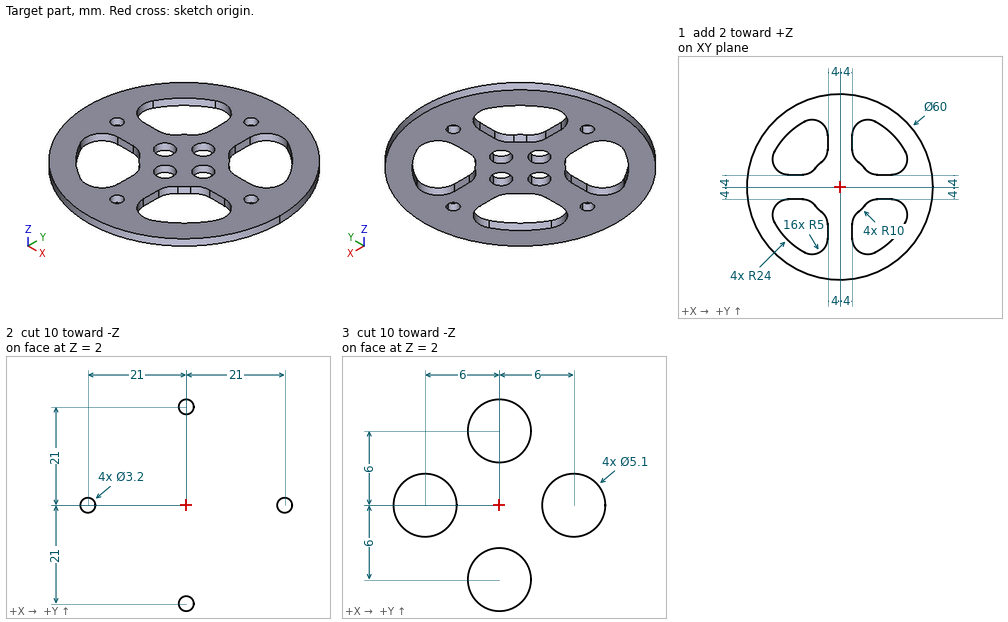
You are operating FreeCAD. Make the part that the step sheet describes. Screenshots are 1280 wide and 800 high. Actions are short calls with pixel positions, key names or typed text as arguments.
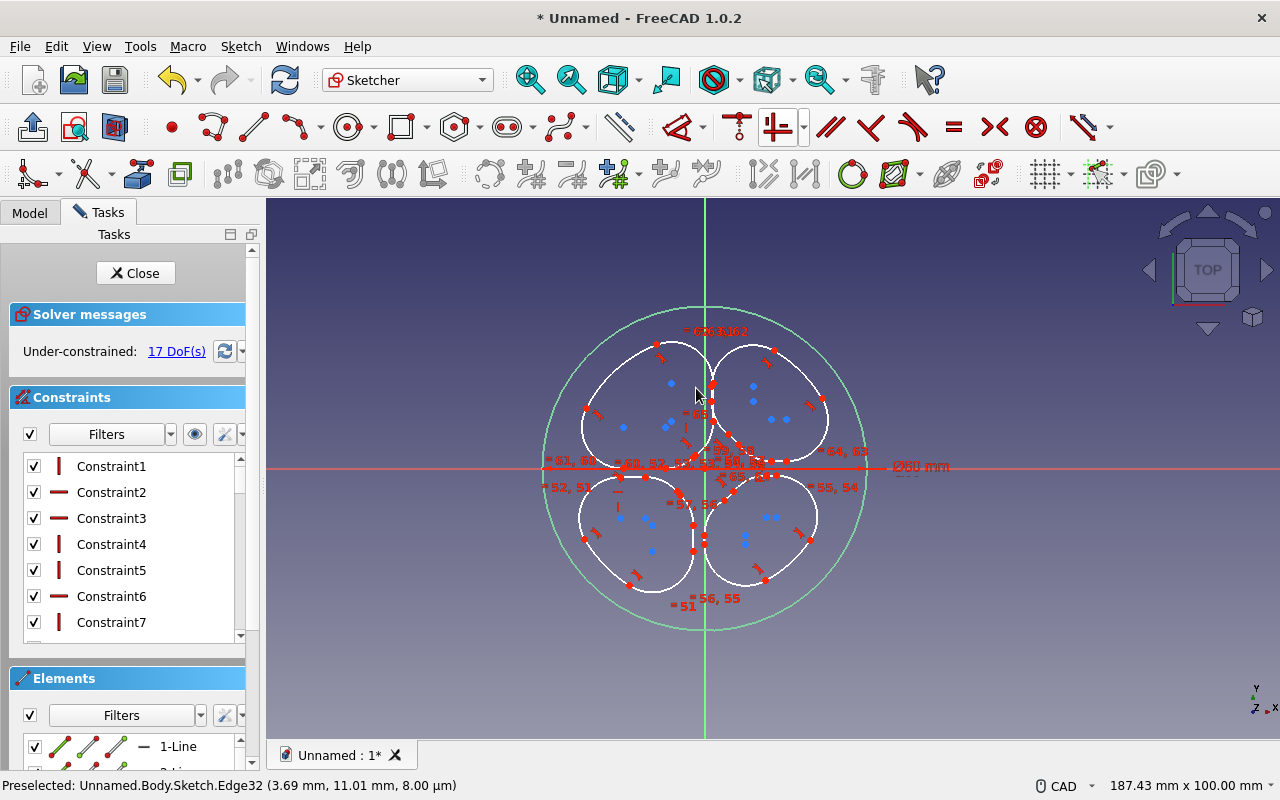
click(596, 556)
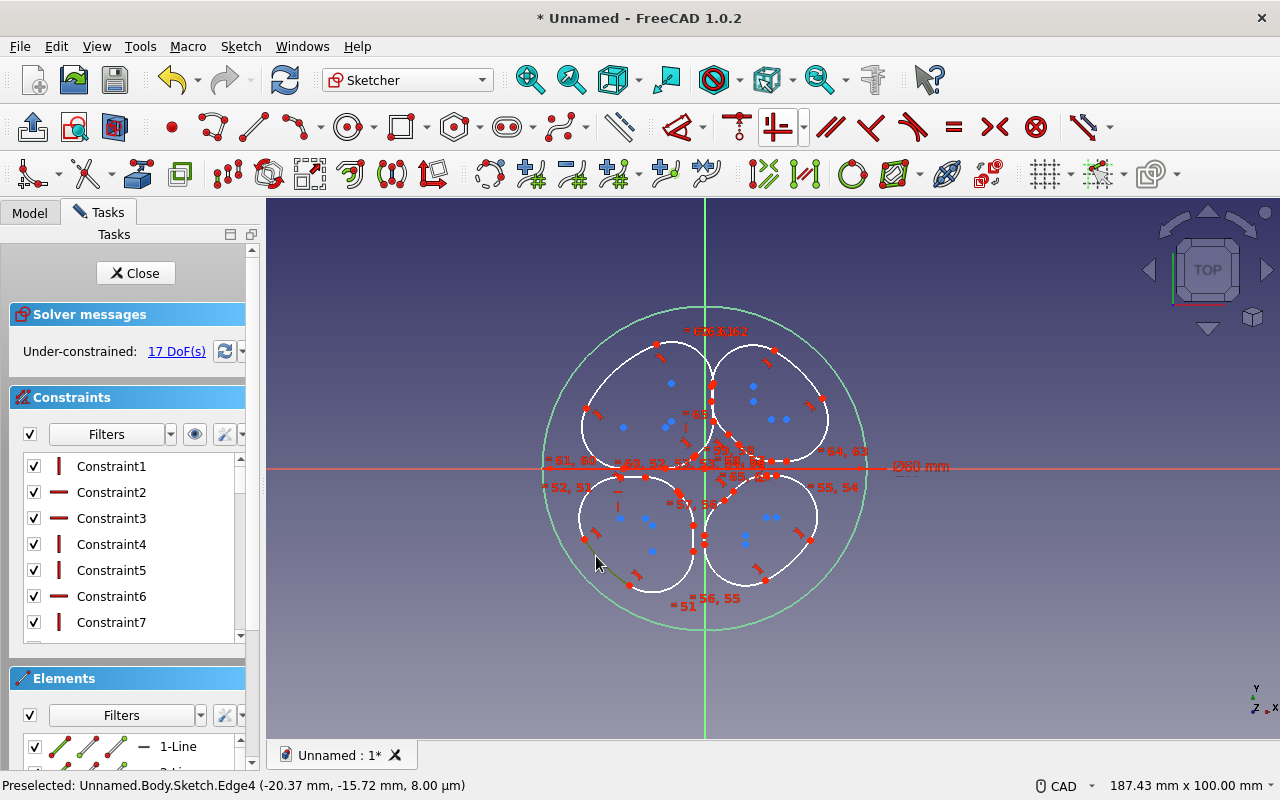
click(781, 571)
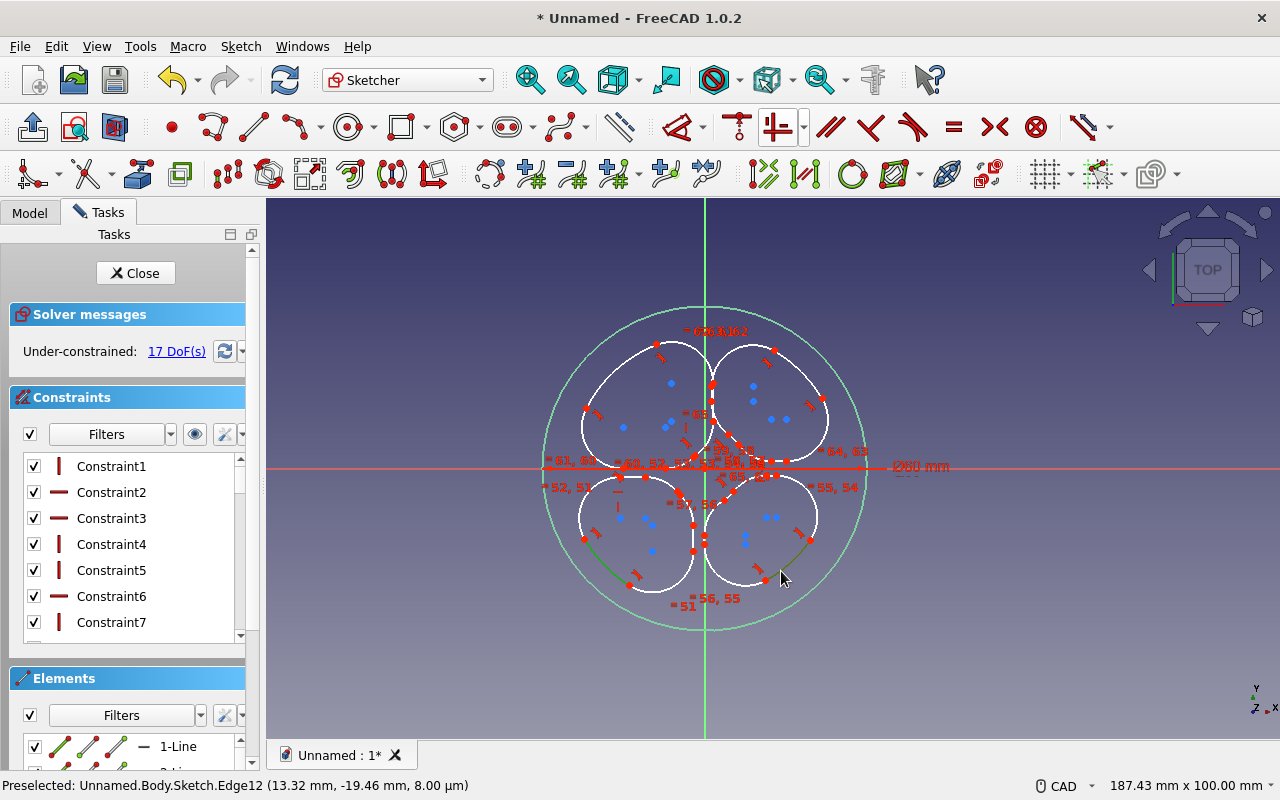
click(631, 358)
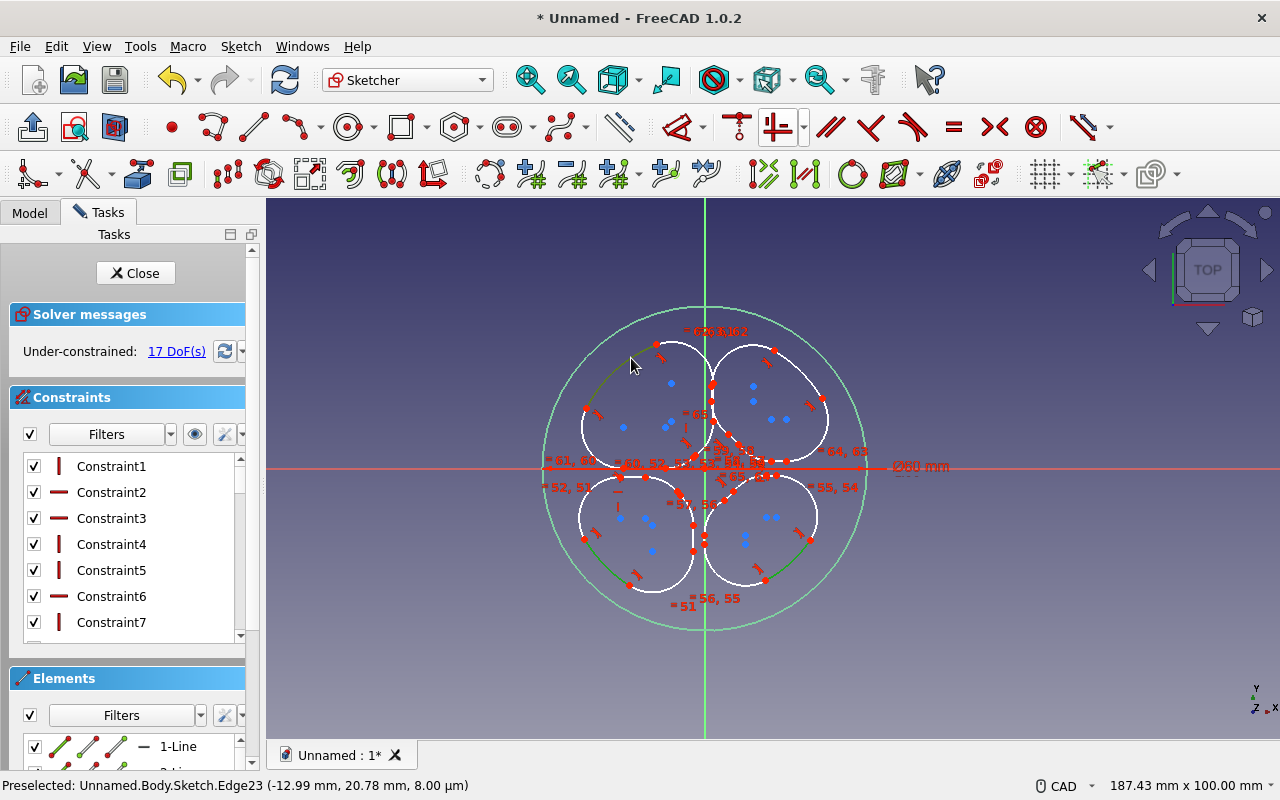
click(810, 382)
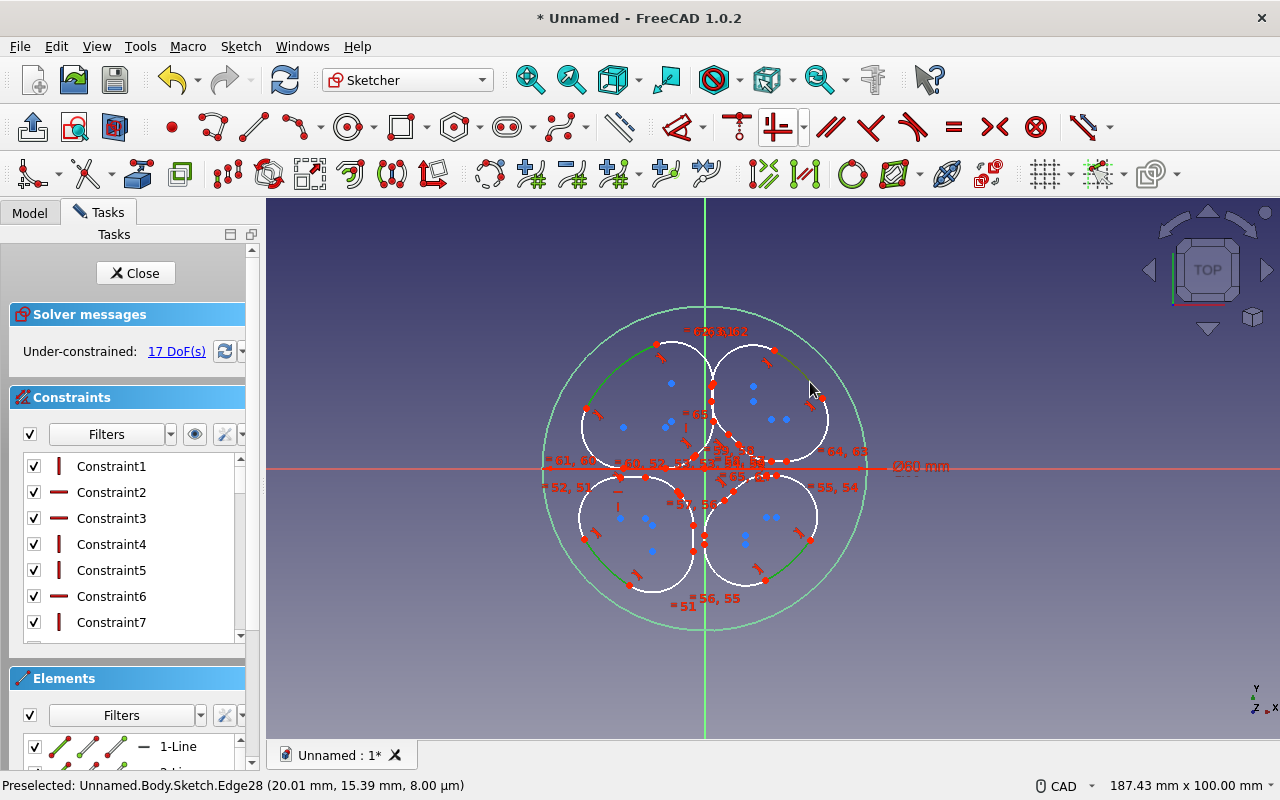
key(e)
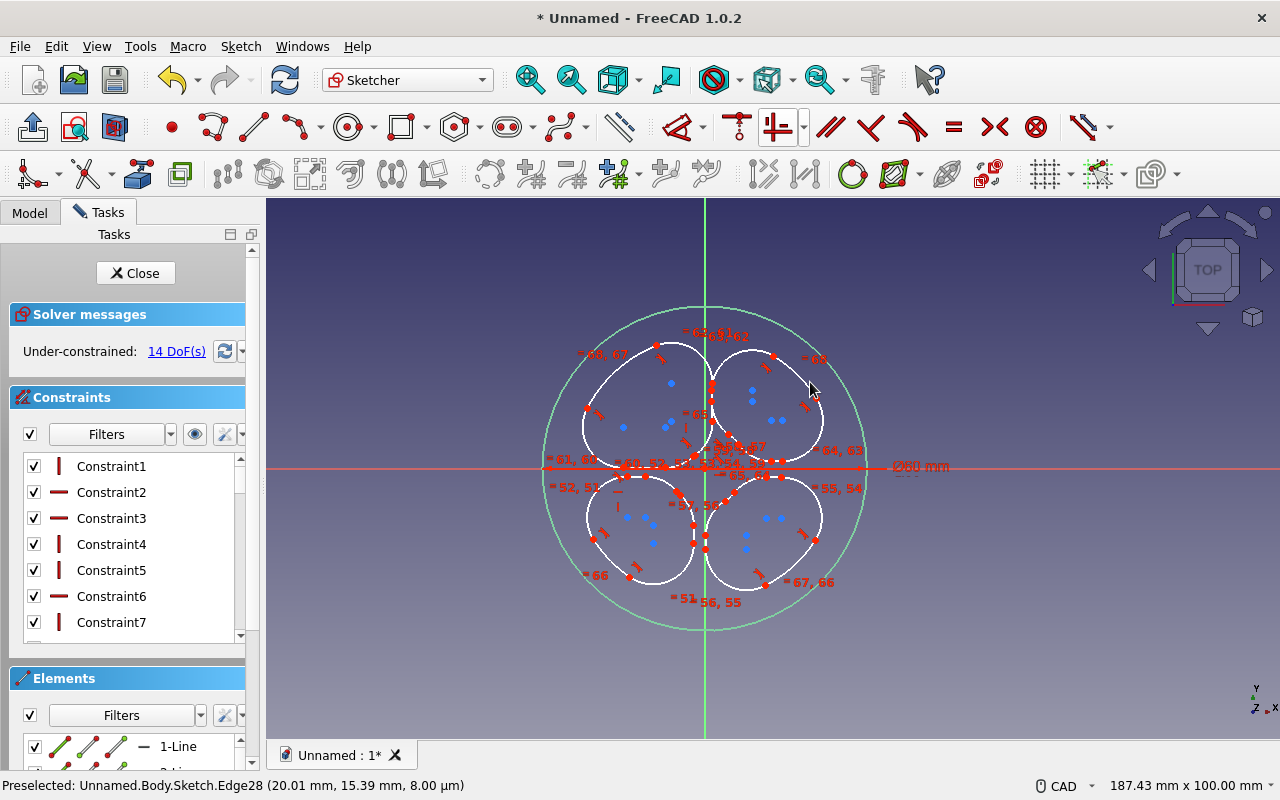
scroll(679, 493, up, 9)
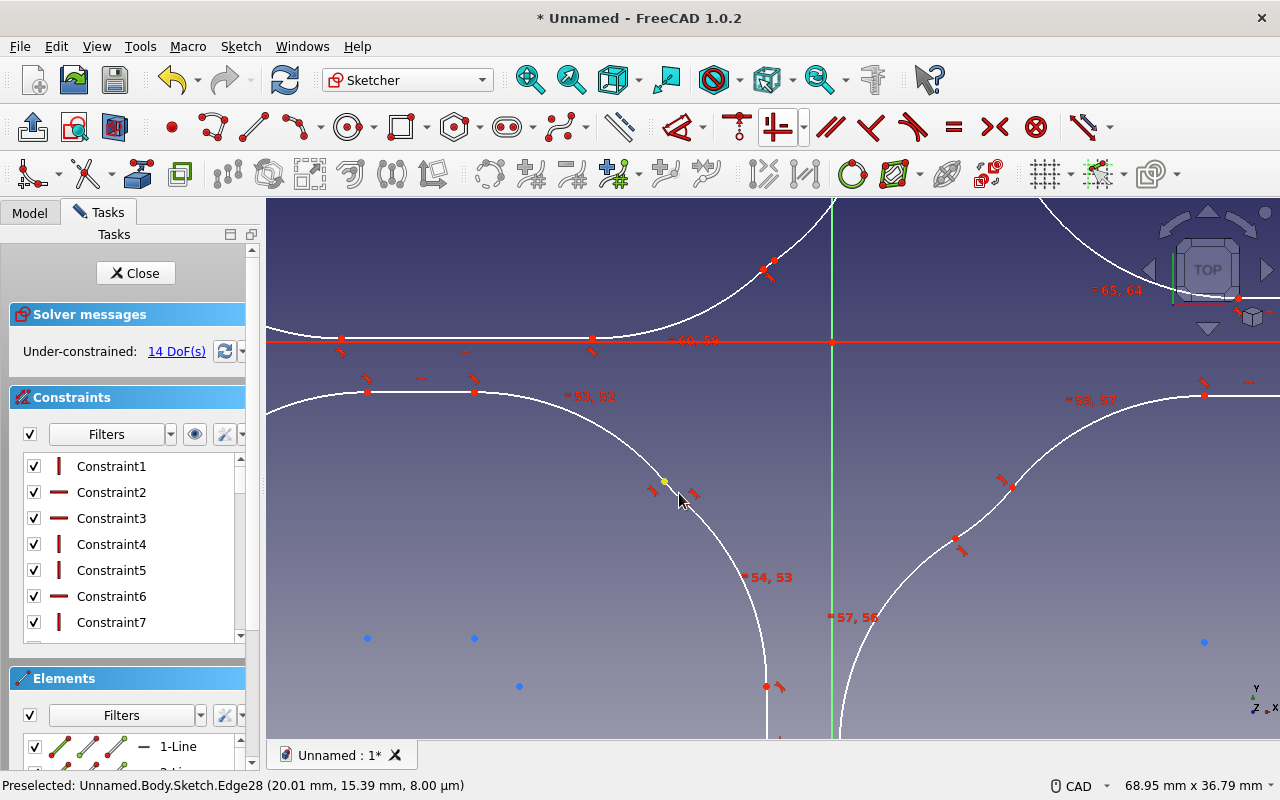
click(675, 493)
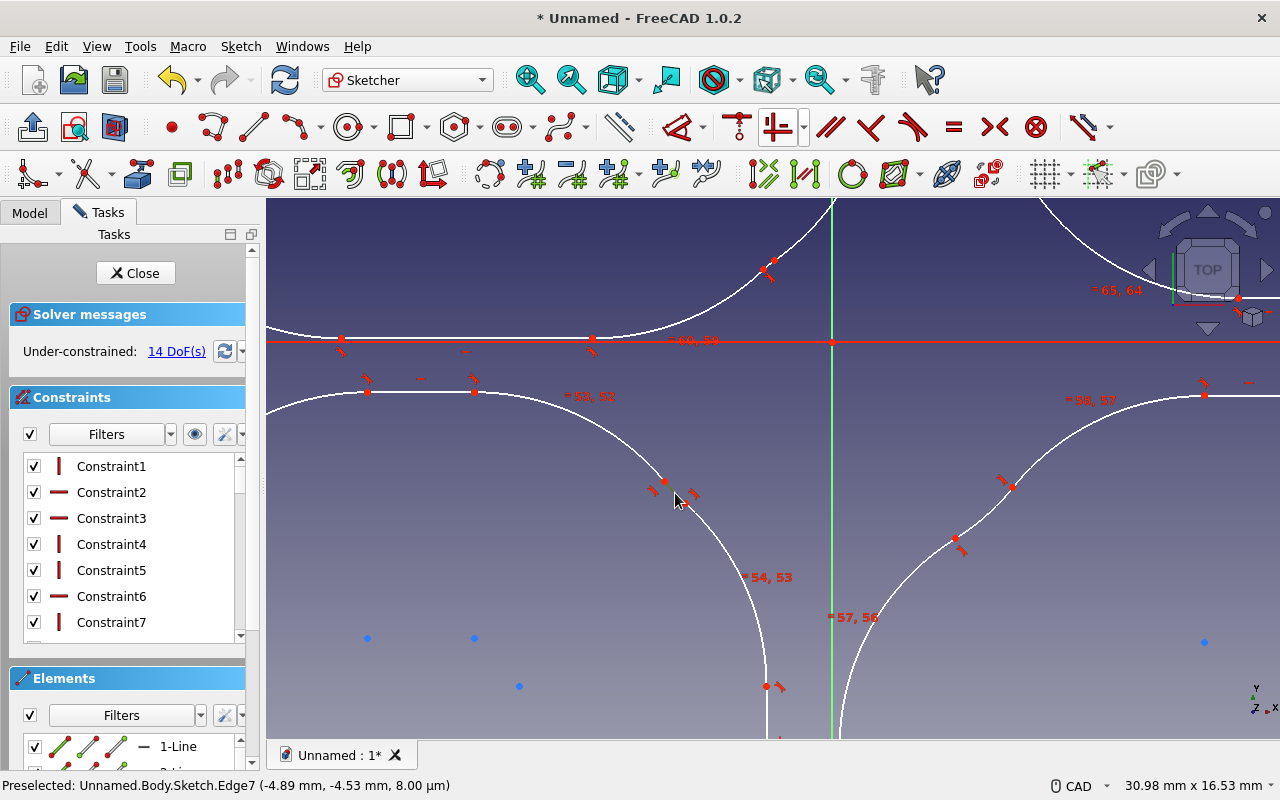
click(974, 525)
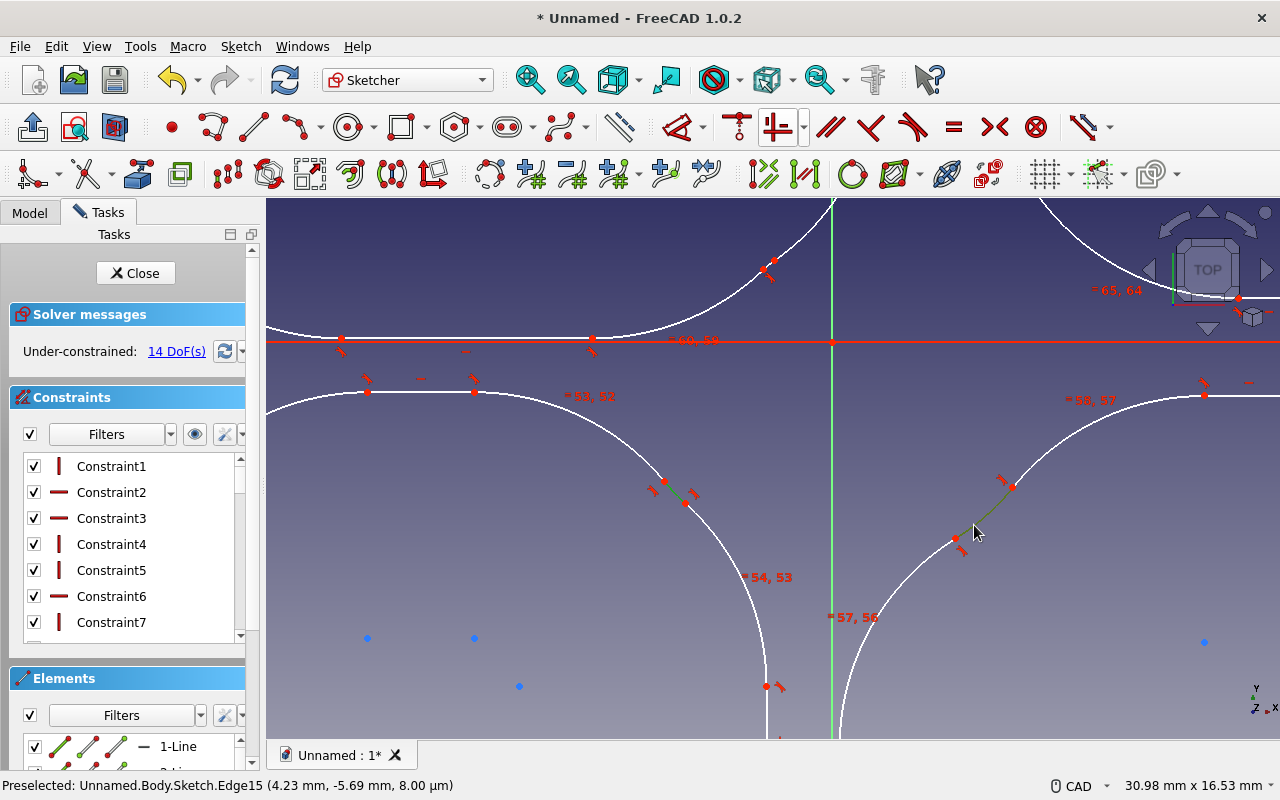
scroll(769, 265, up, 4)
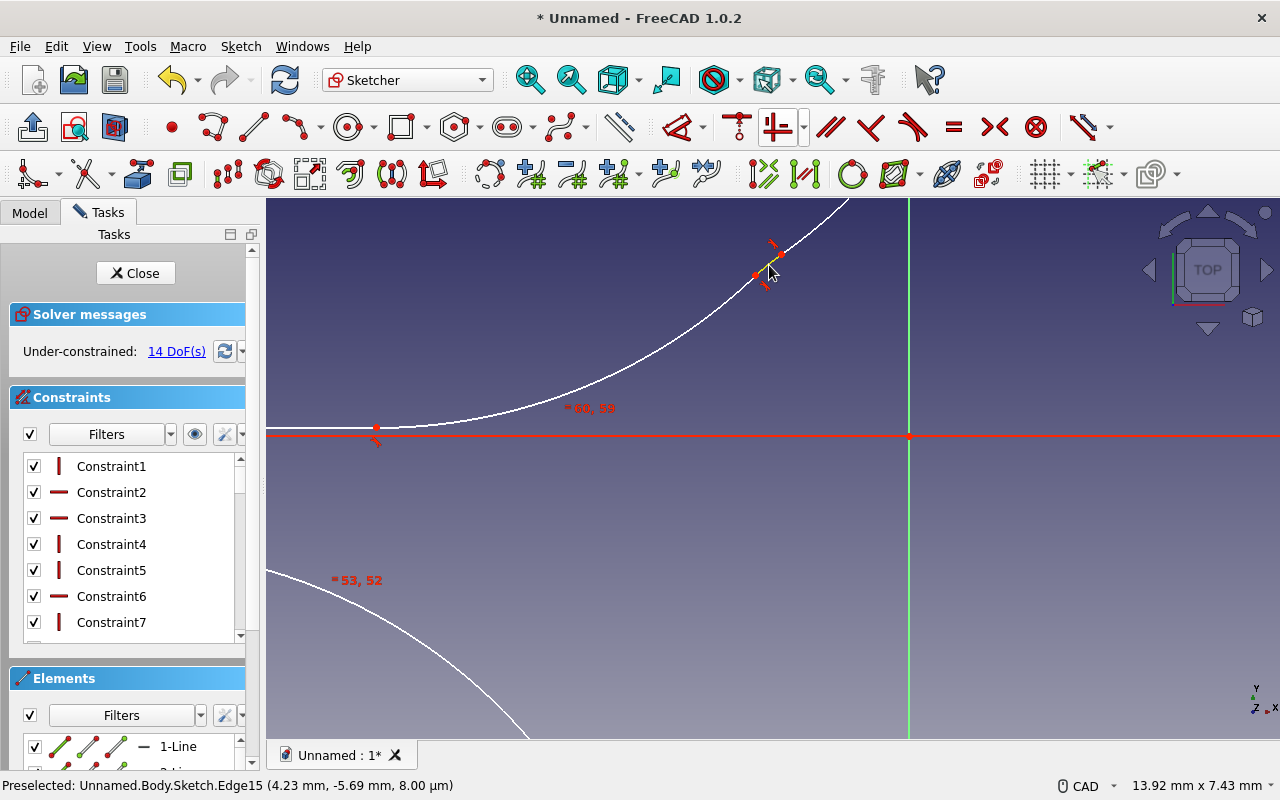
click(768, 265)